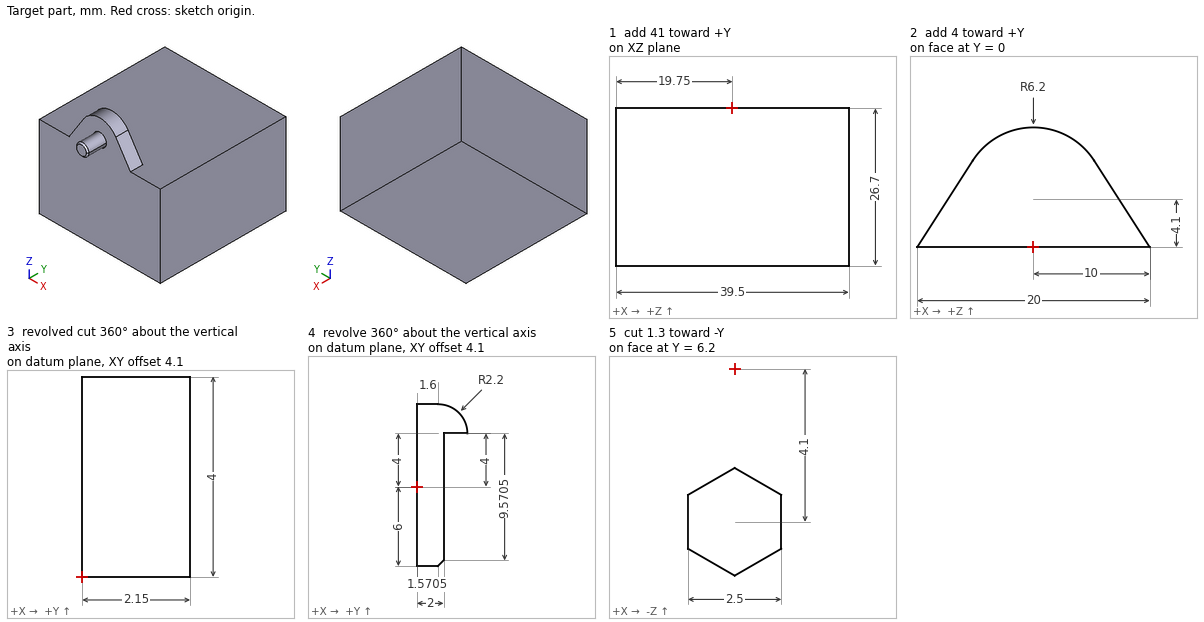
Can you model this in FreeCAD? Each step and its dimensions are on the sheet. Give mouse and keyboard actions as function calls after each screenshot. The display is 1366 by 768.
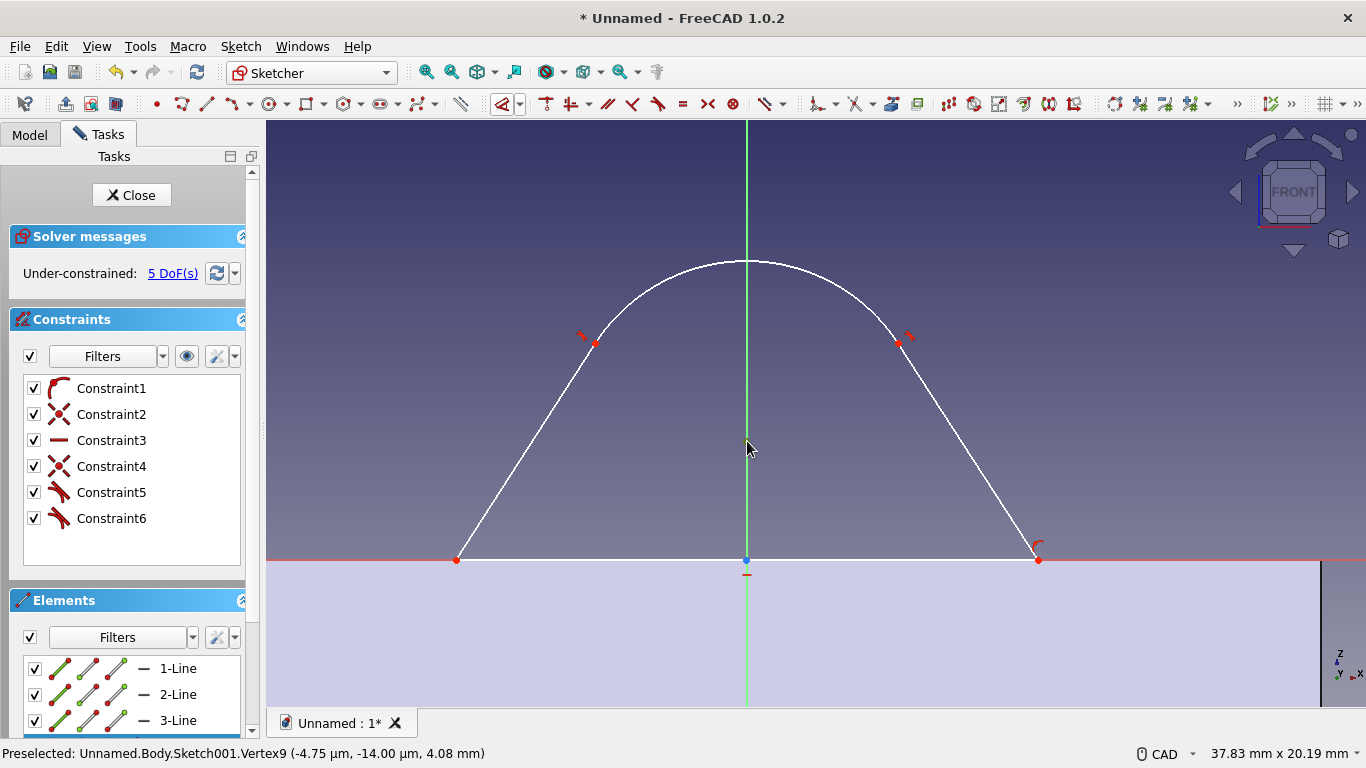
click(747, 641)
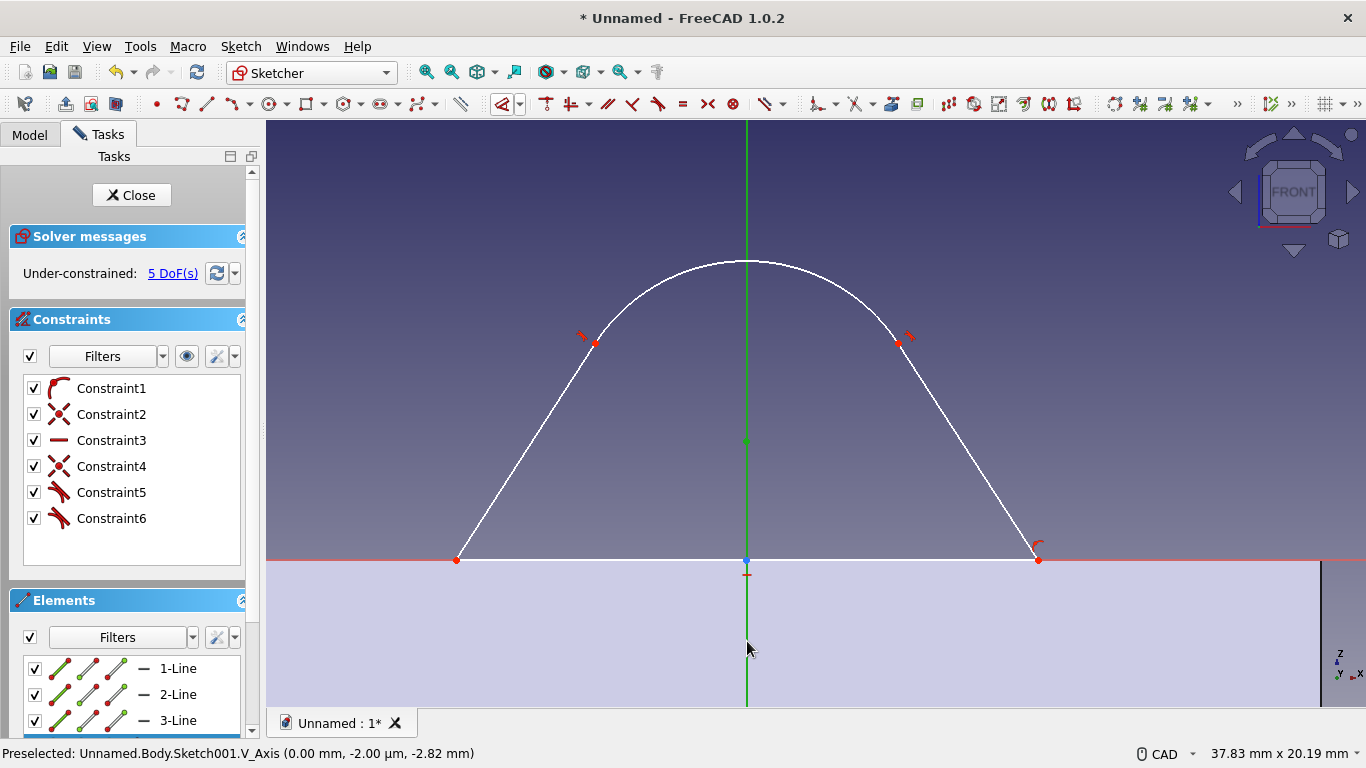
key(c)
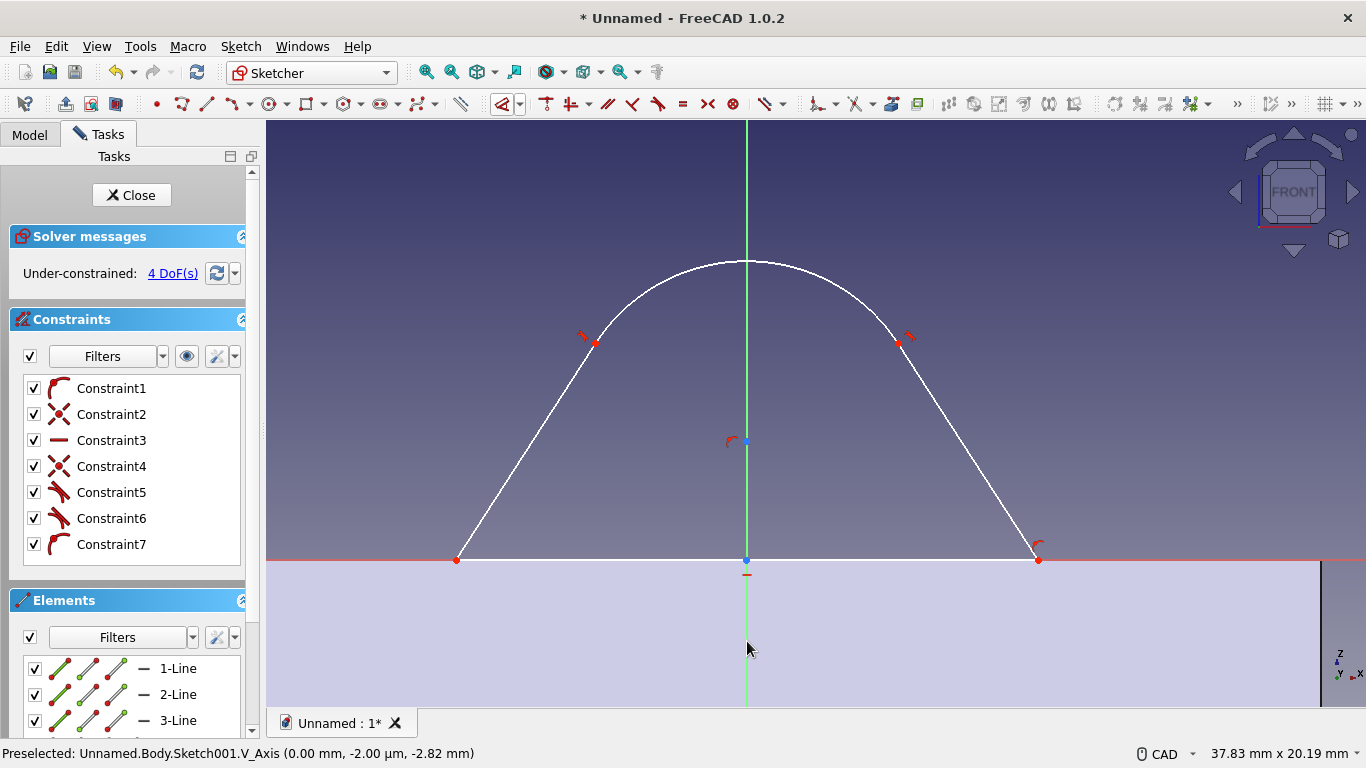
click(817, 275)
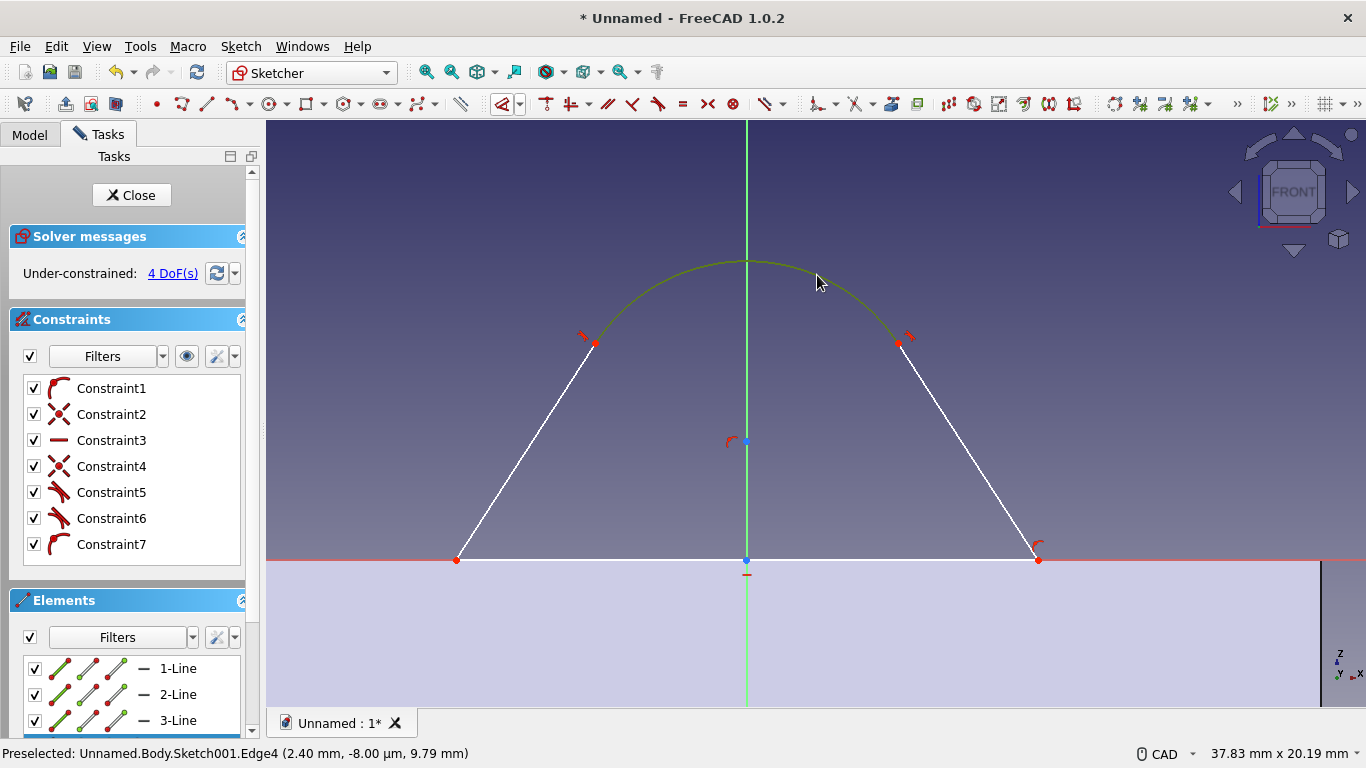
key(k)
key(r)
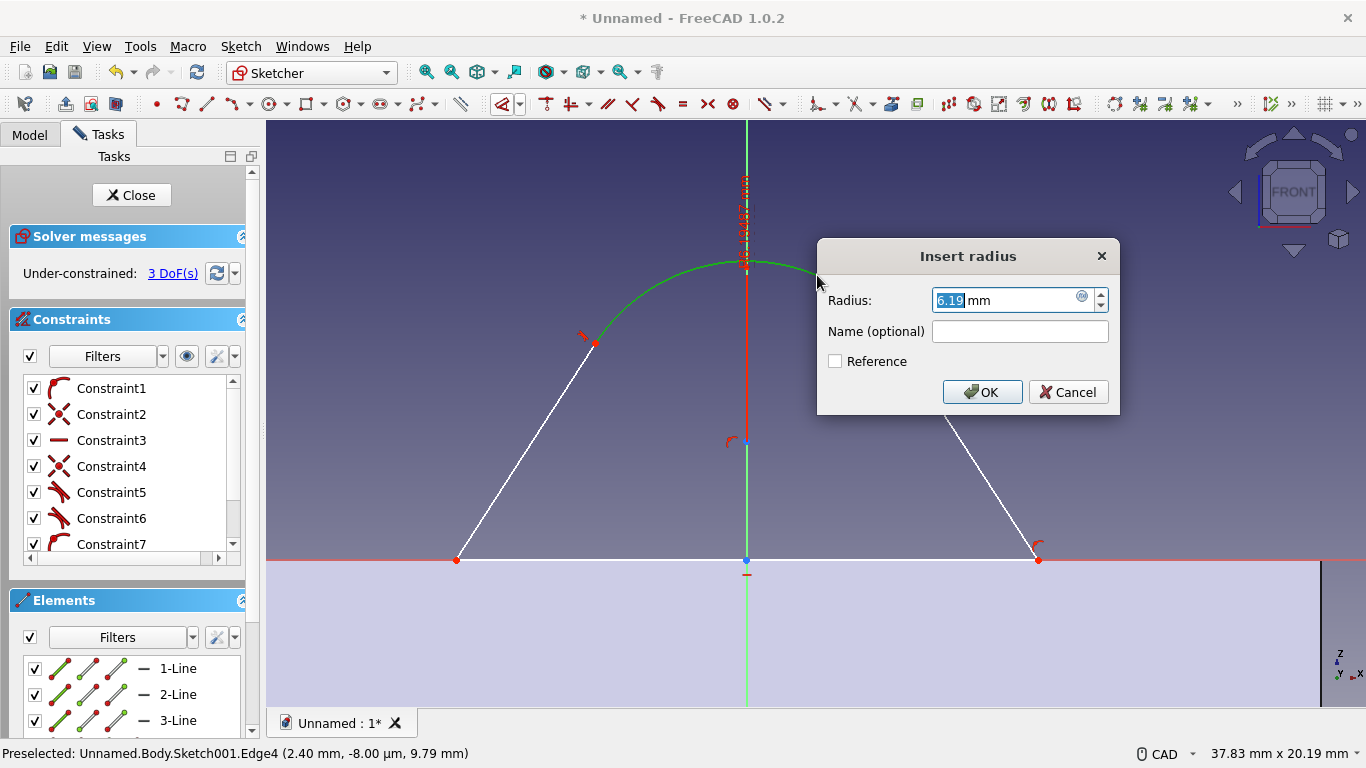
text(6.2)
key(Return)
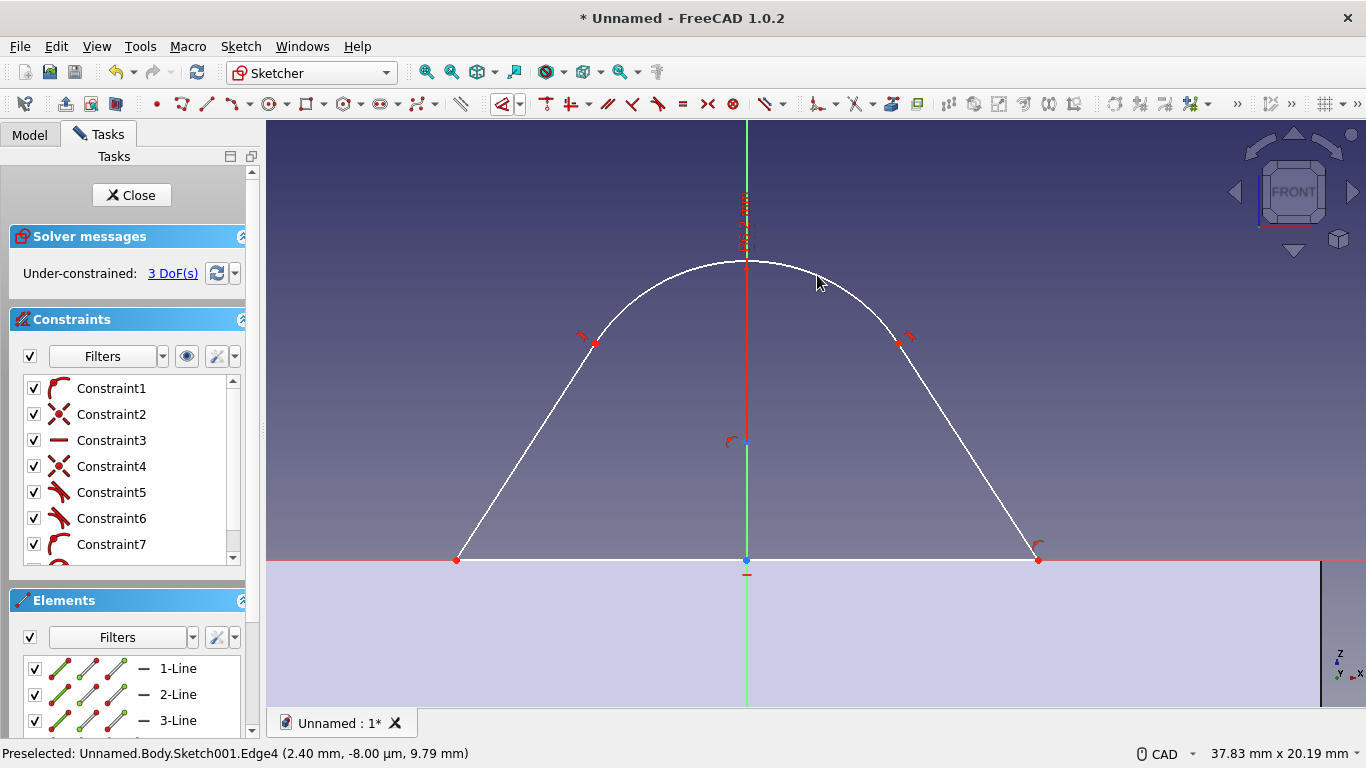
click(863, 560)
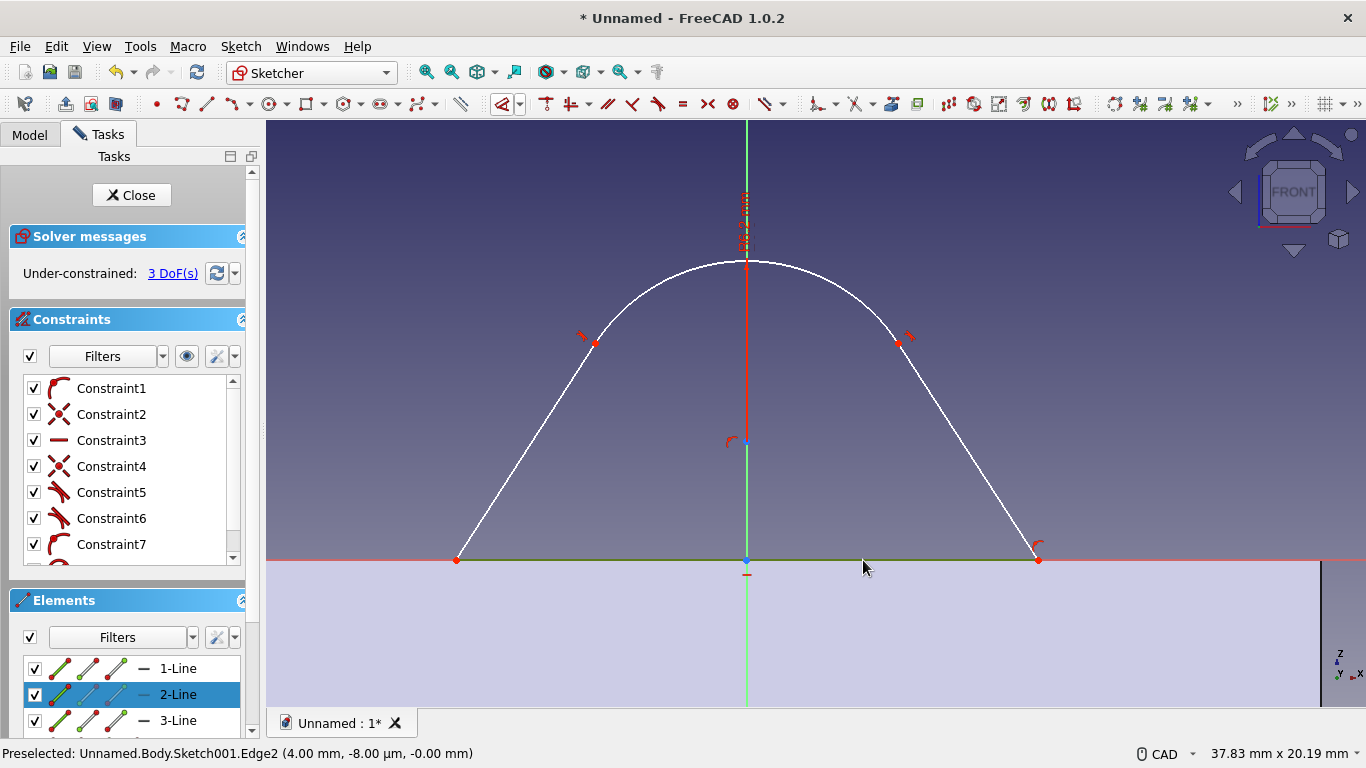
key(l)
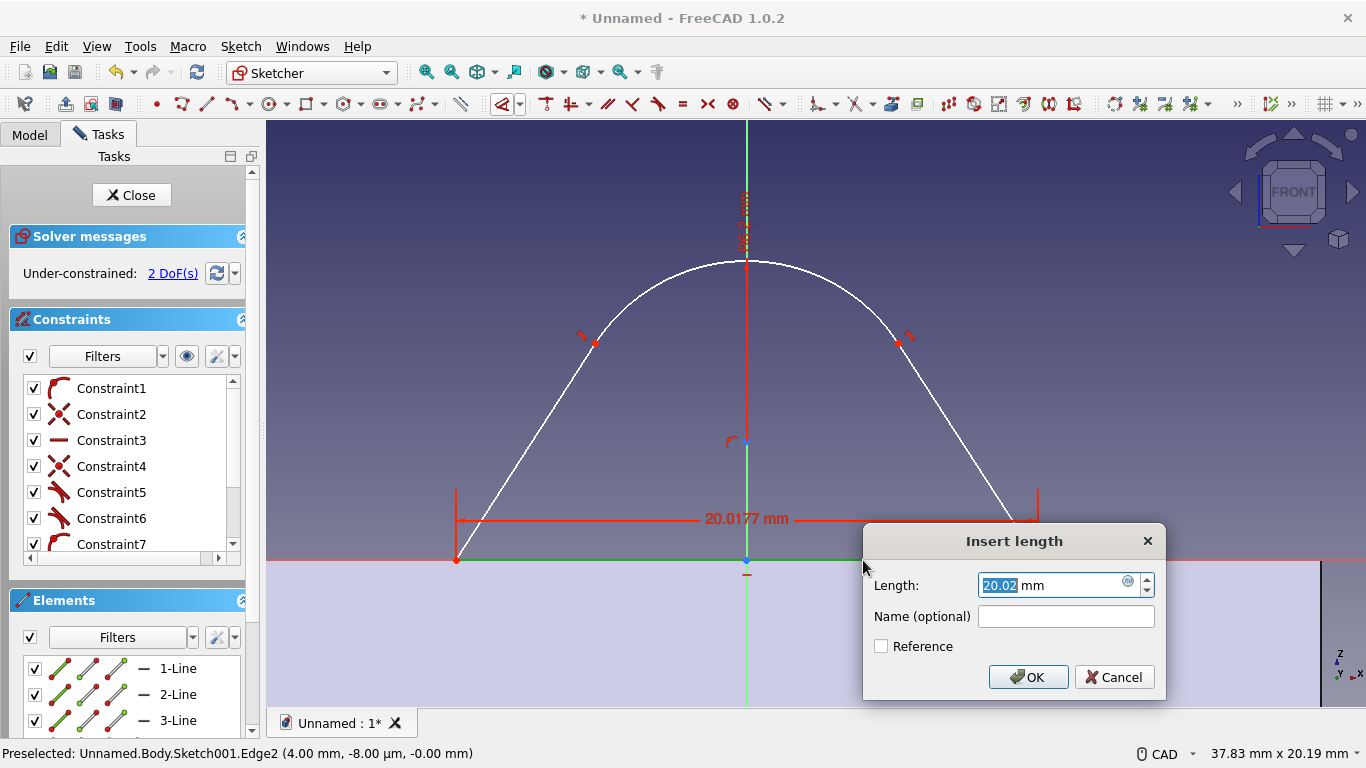
text(20)
key(Return)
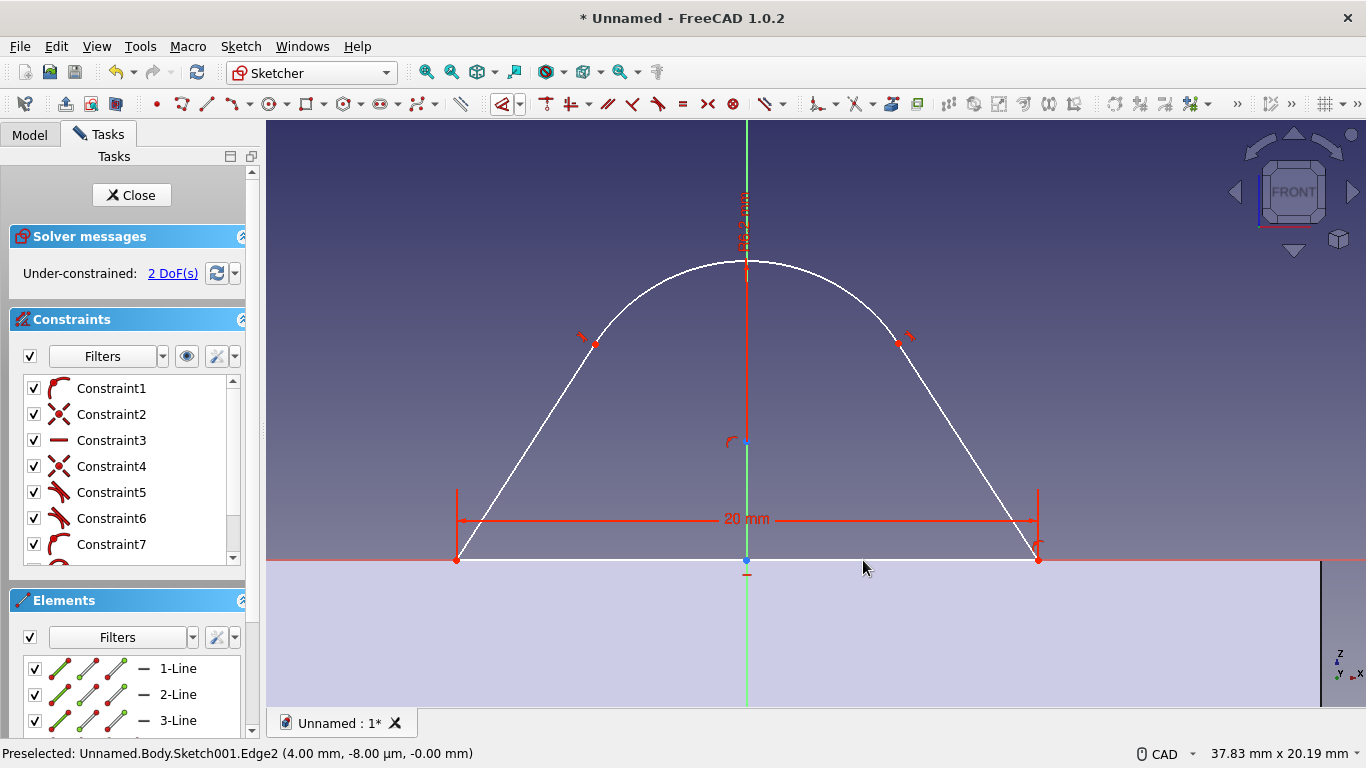
click(1038, 560)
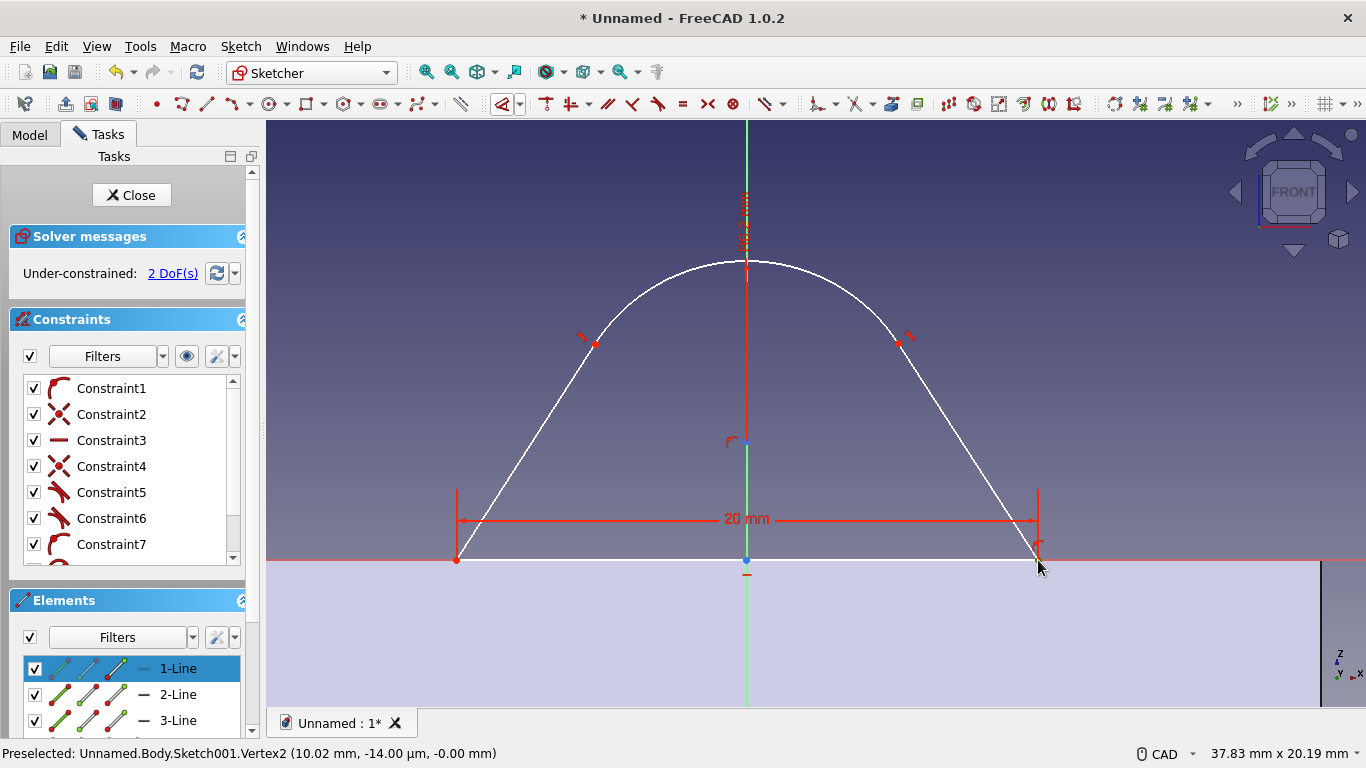
key(l)